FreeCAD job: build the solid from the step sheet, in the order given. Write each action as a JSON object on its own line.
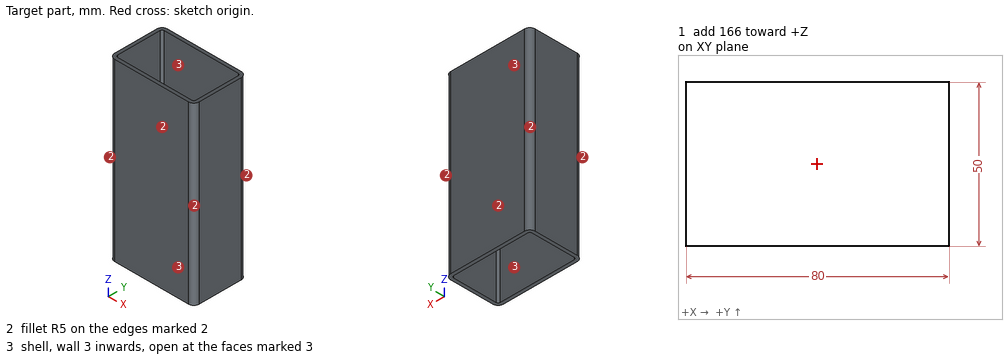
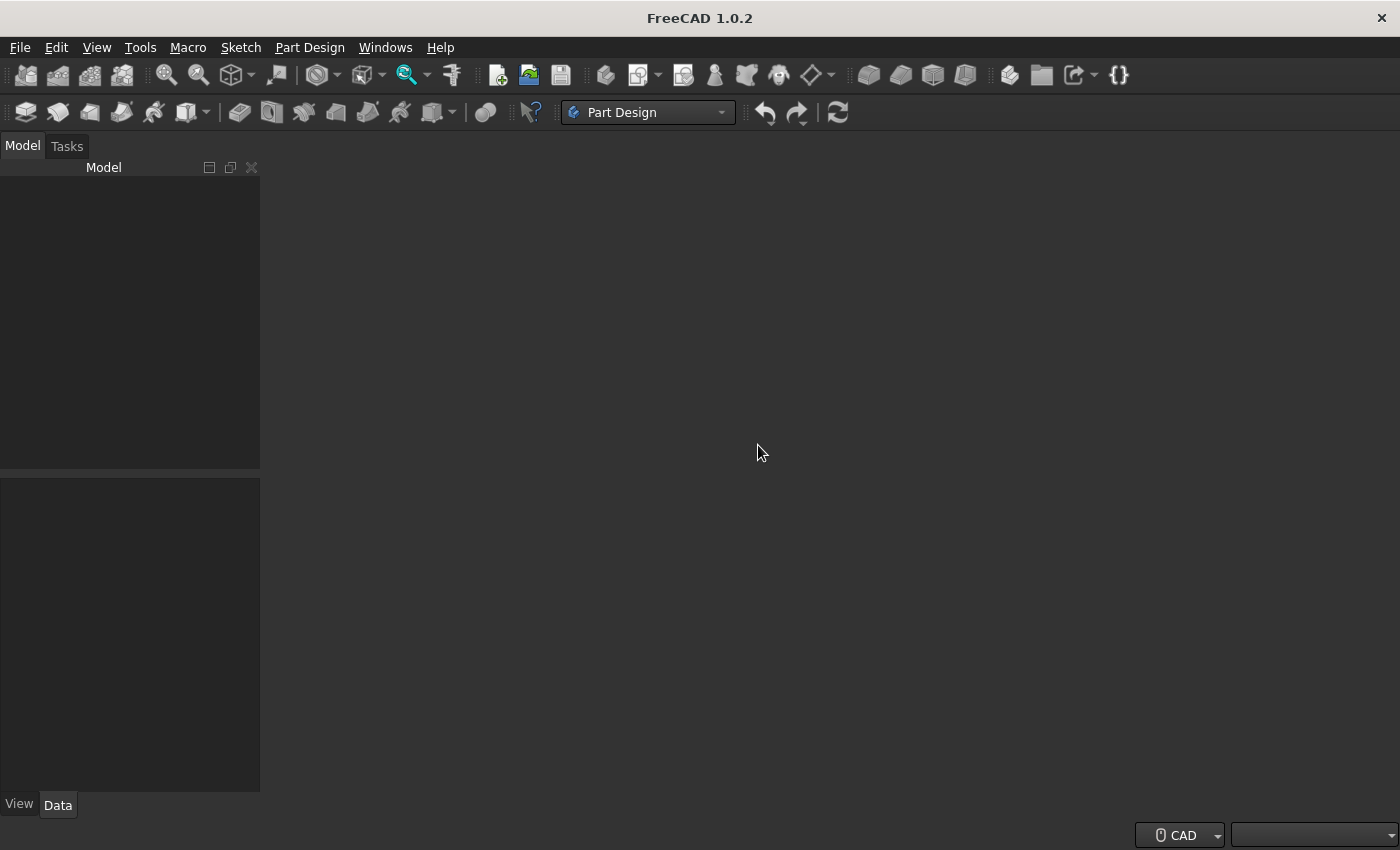
{"action": "left_click", "coordinate": [498, 76]}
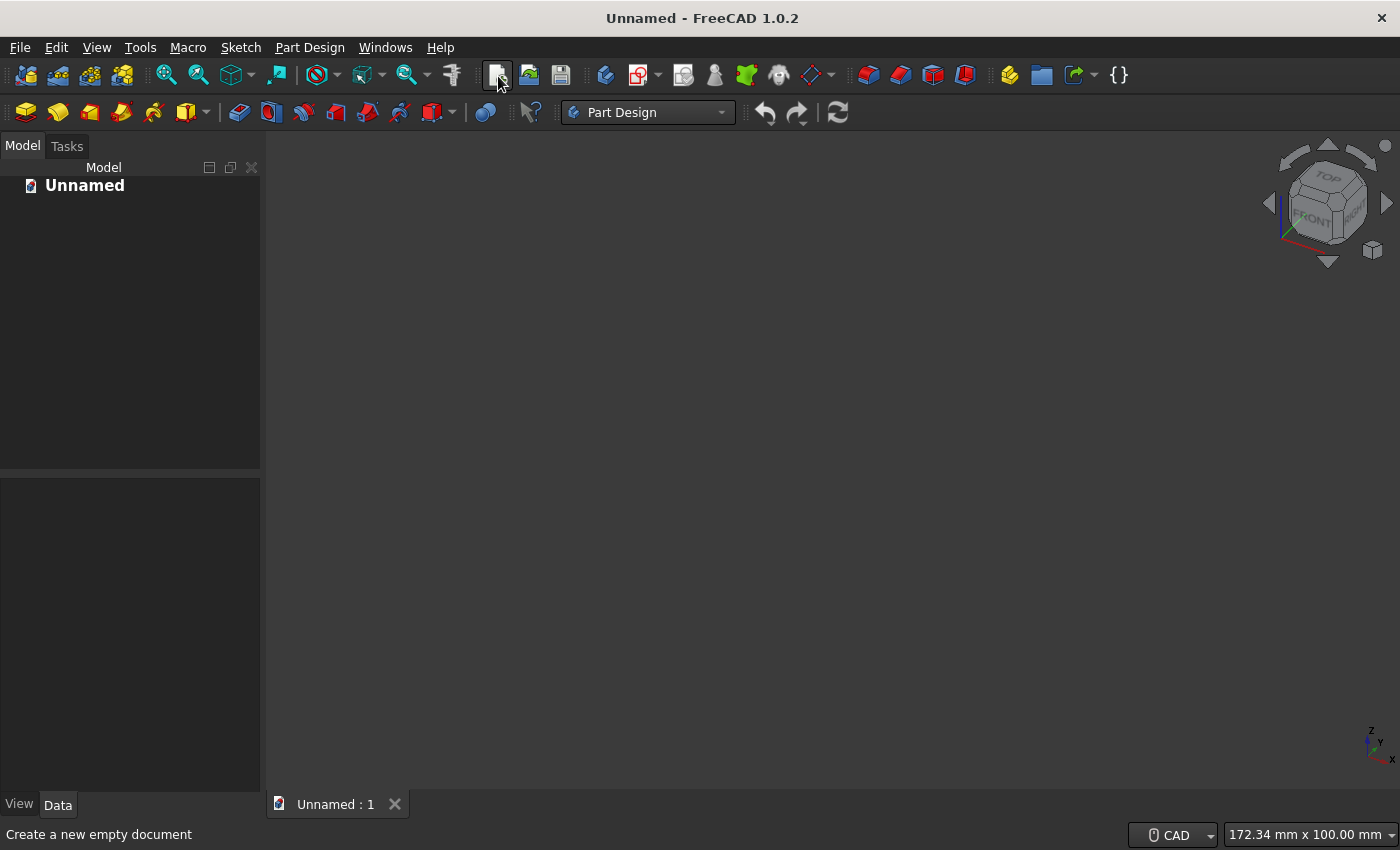
{"action": "left_click", "coordinate": [638, 76]}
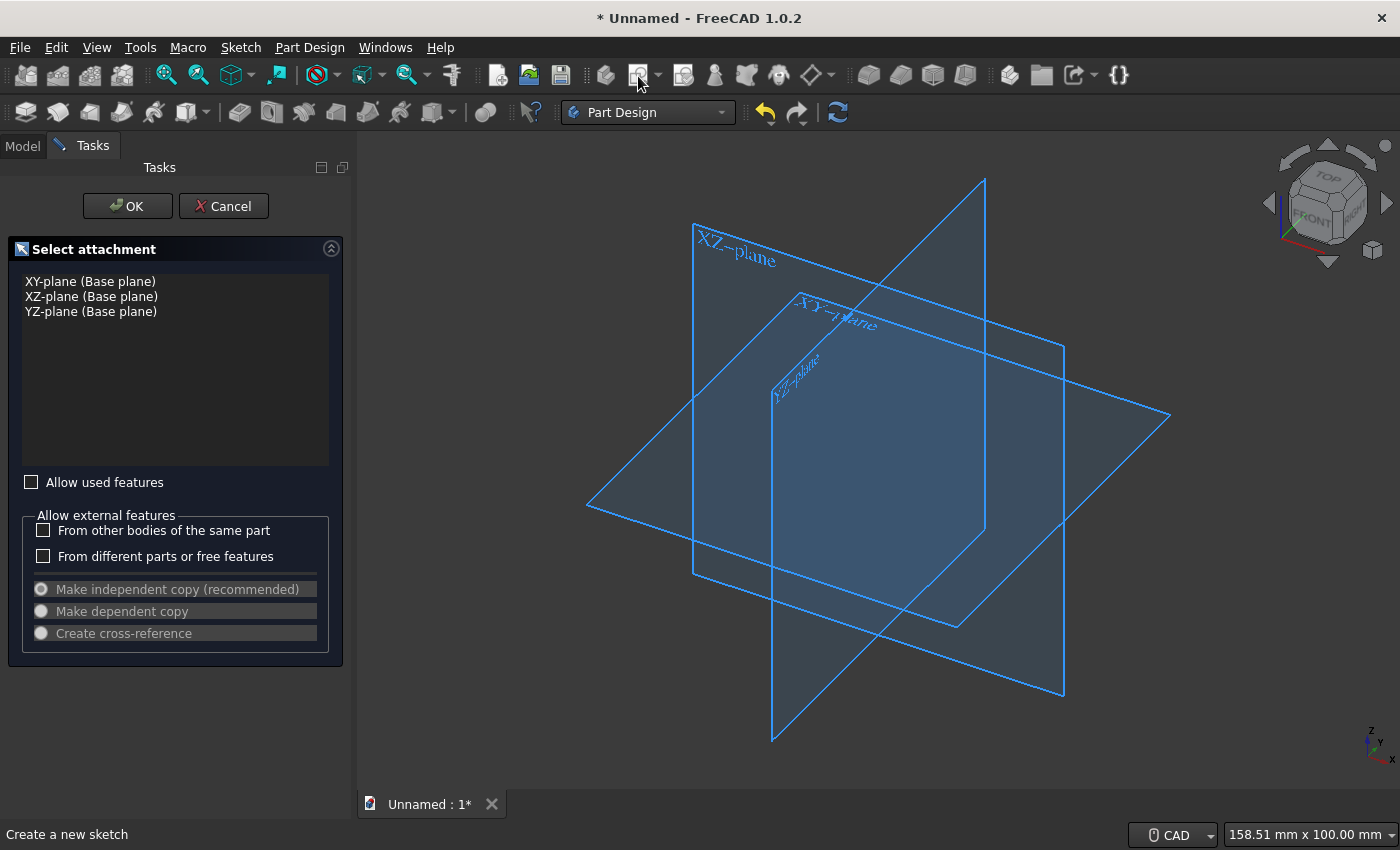
{"action": "left_click", "coordinate": [82, 282]}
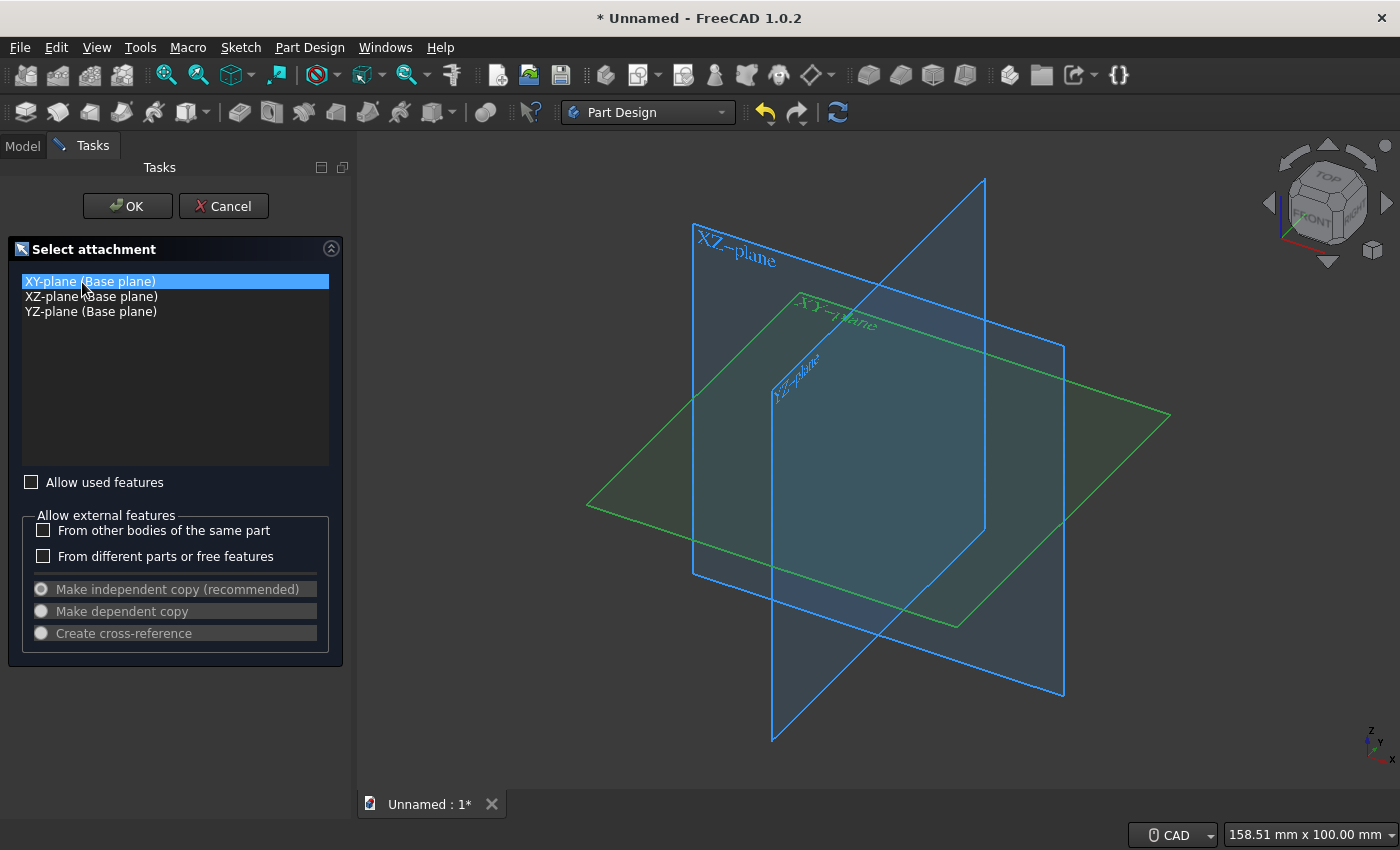
{"action": "left_click", "coordinate": [128, 206]}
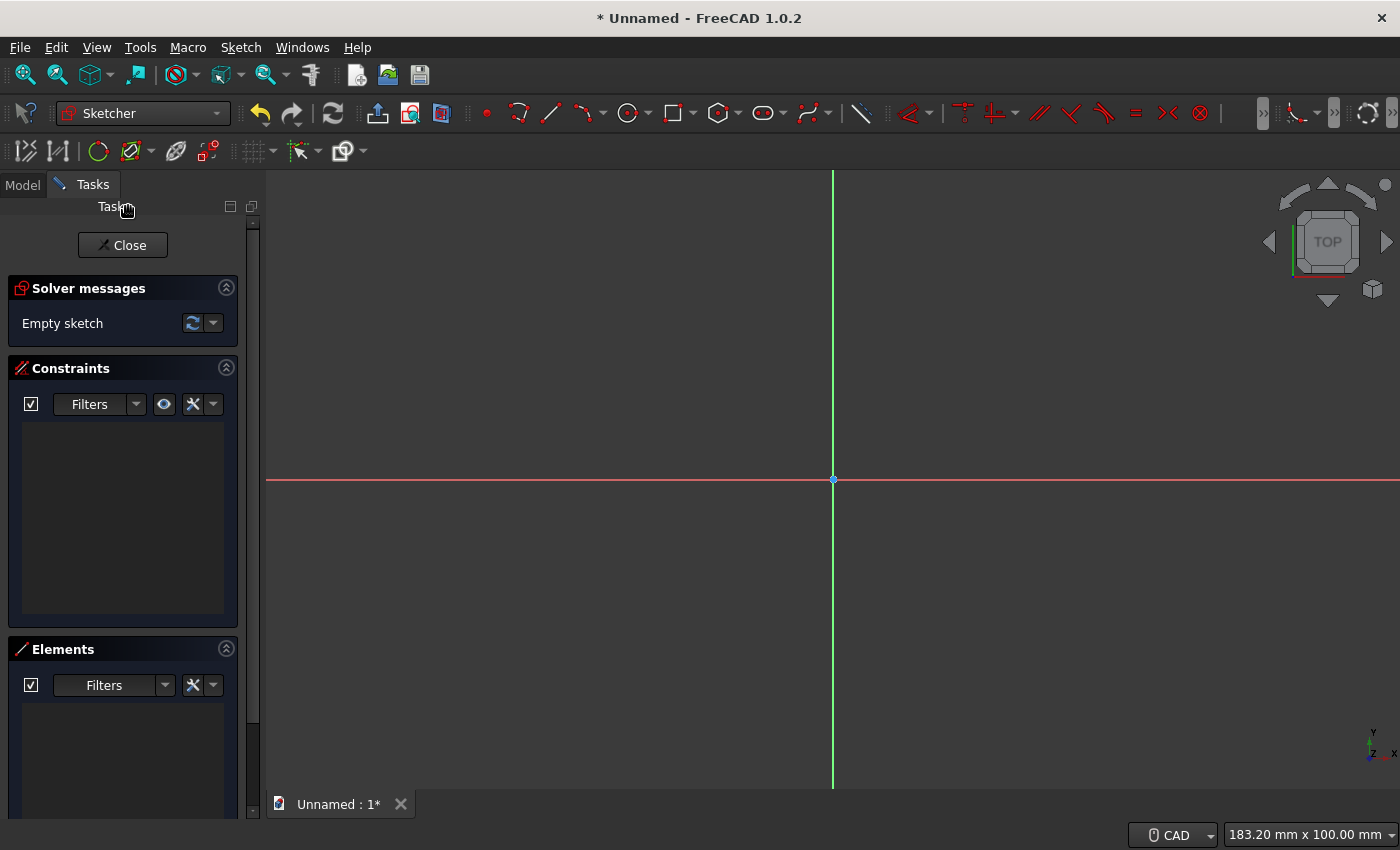
{"action": "key", "text": "g v"}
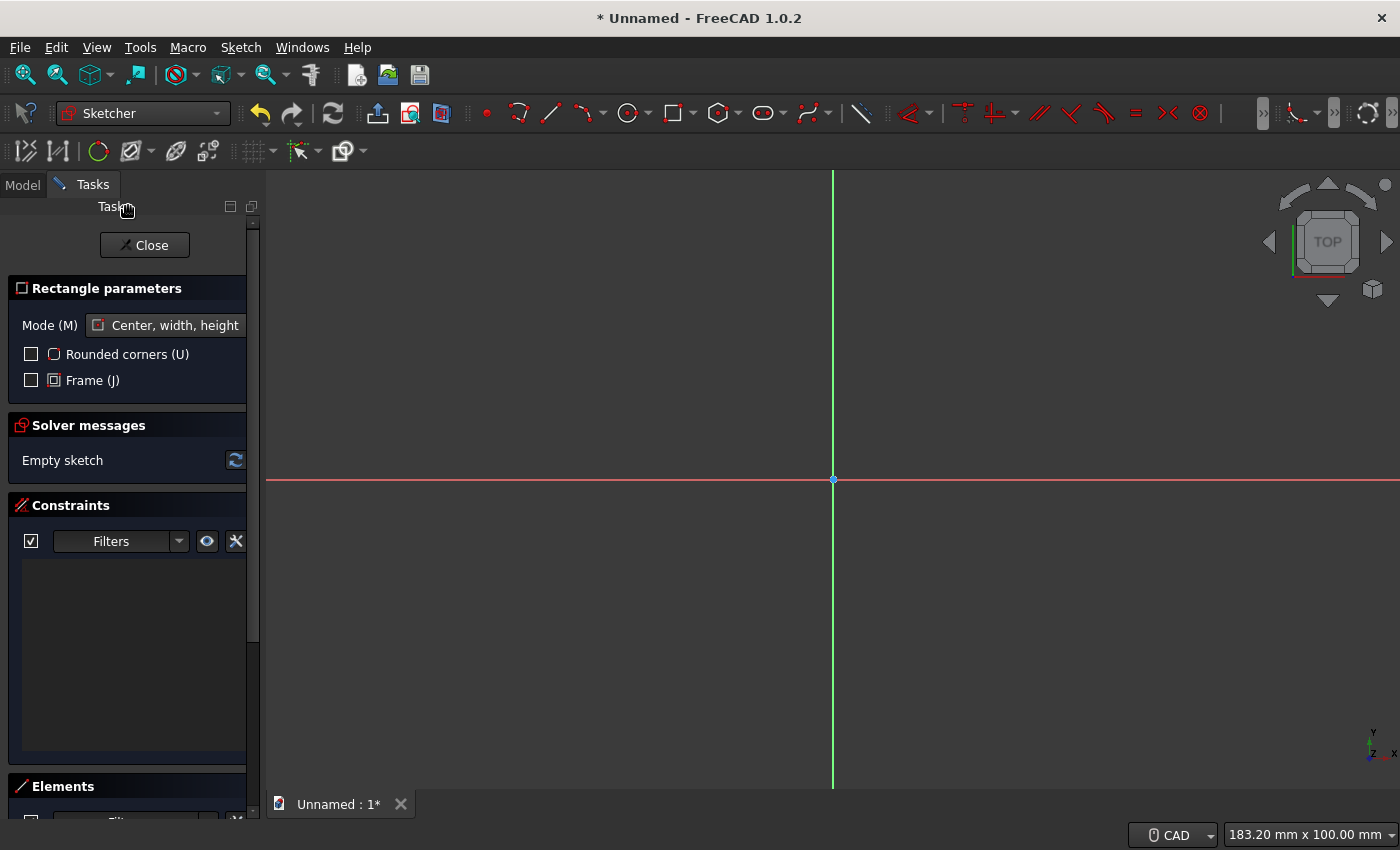
{"action": "left_click", "coordinate": [833, 480]}
{"action": "left_click", "coordinate": [1081, 325]}
{"action": "key", "text": "Escape"}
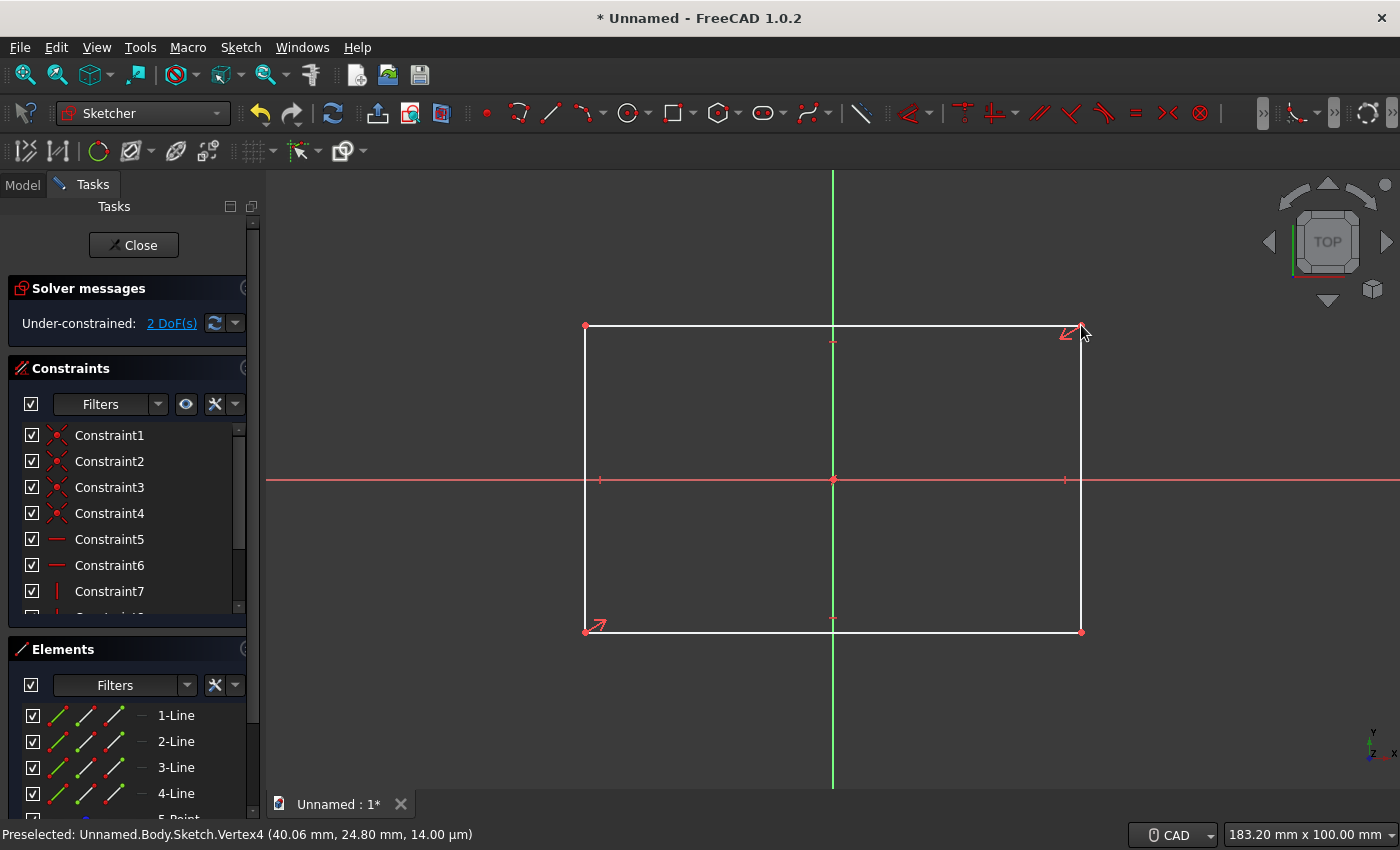
{"action": "key", "text": "d"}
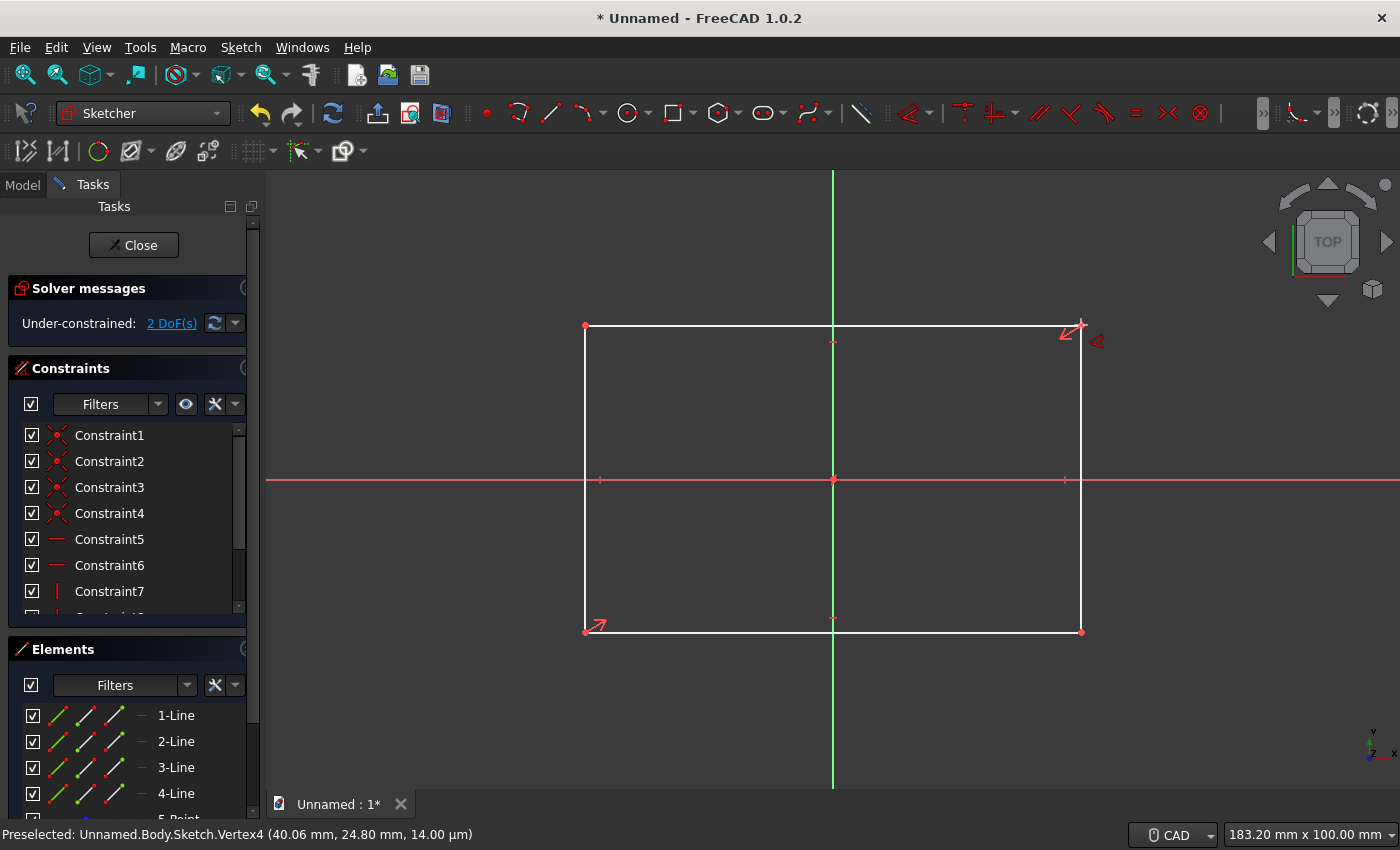
{"action": "left_click", "coordinate": [734, 633]}
{"action": "left_click", "coordinate": [719, 667]}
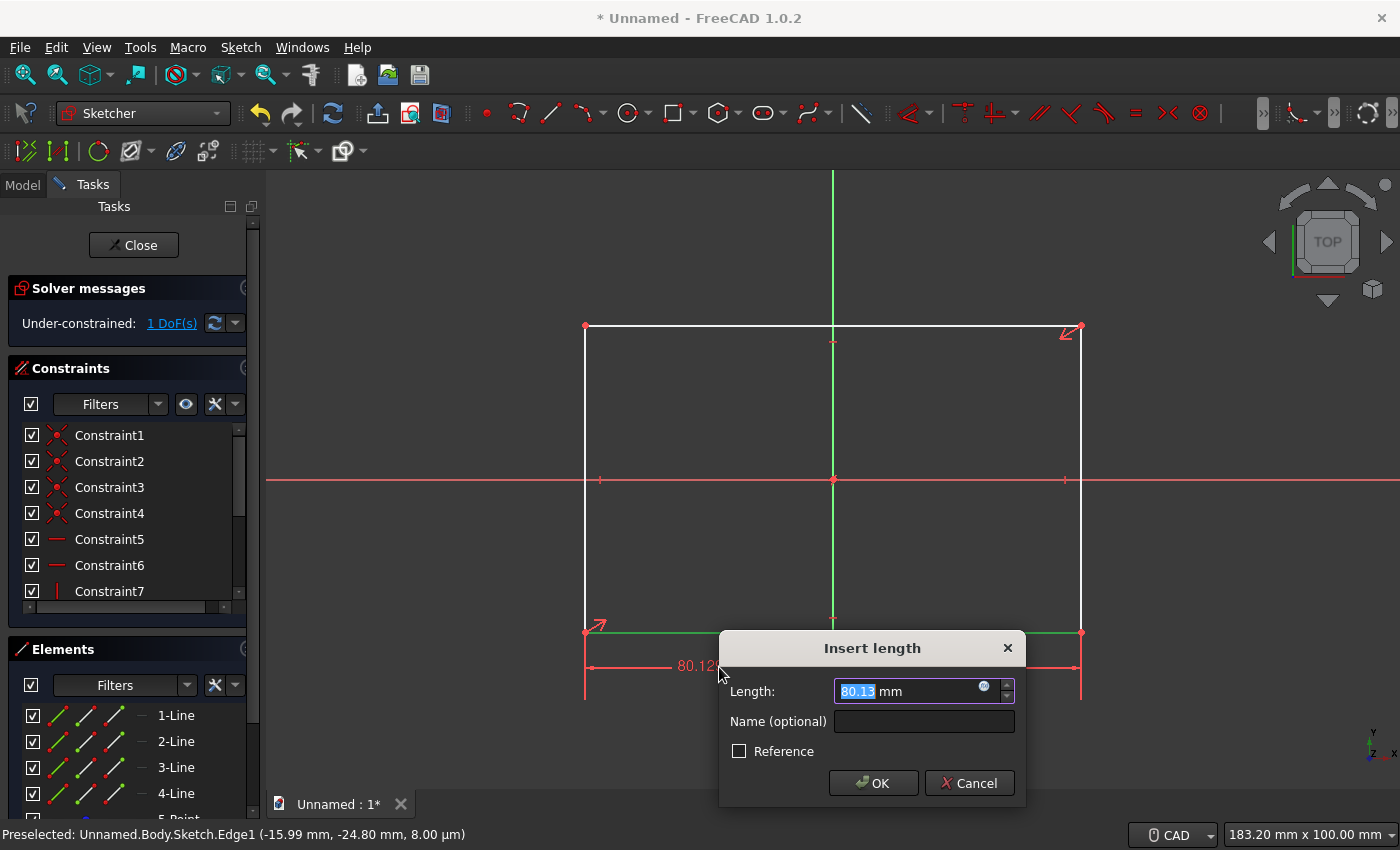
{"action": "type", "text": "80"}
{"action": "key", "text": "Return"}